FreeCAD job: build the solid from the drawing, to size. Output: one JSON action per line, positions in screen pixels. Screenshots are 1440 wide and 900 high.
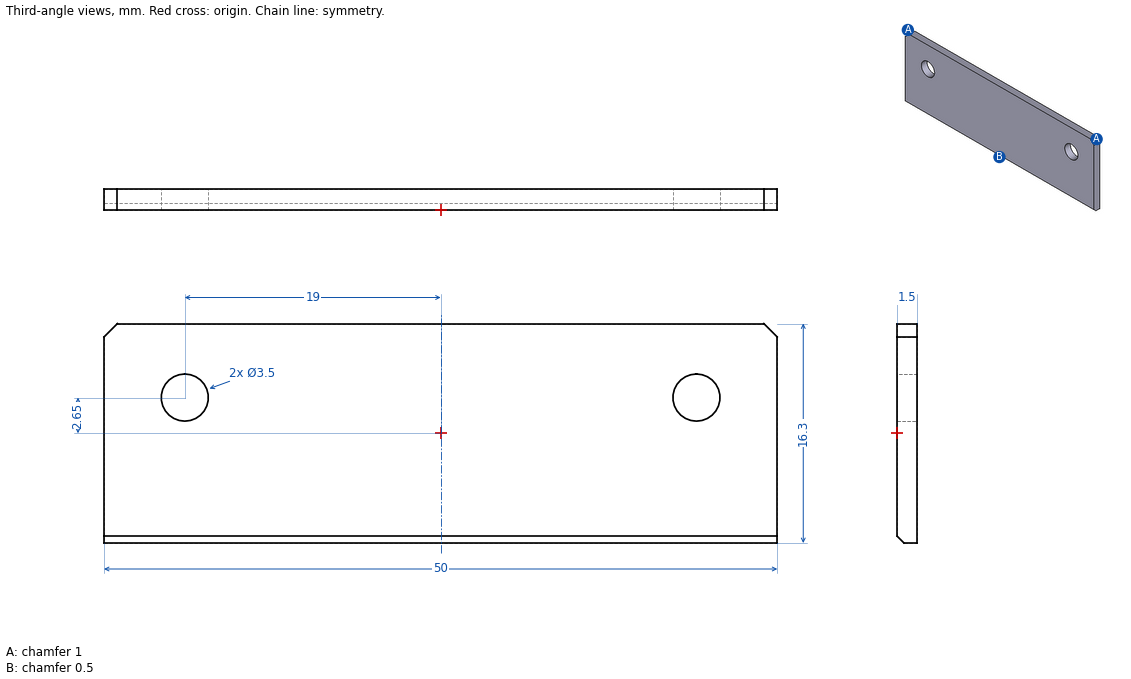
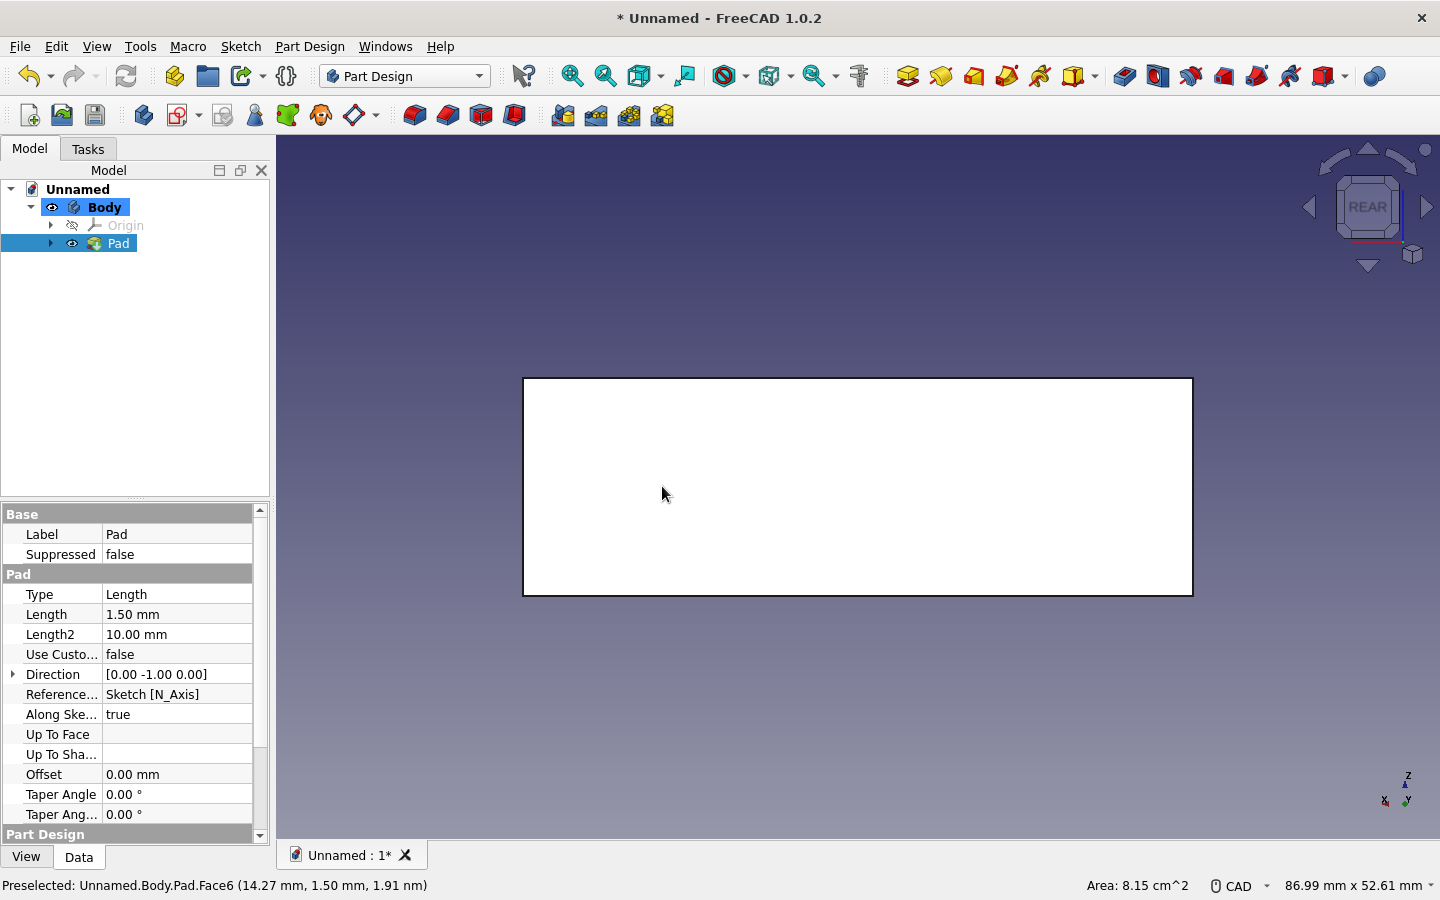
{"action": "left_click", "coordinate": [176, 116]}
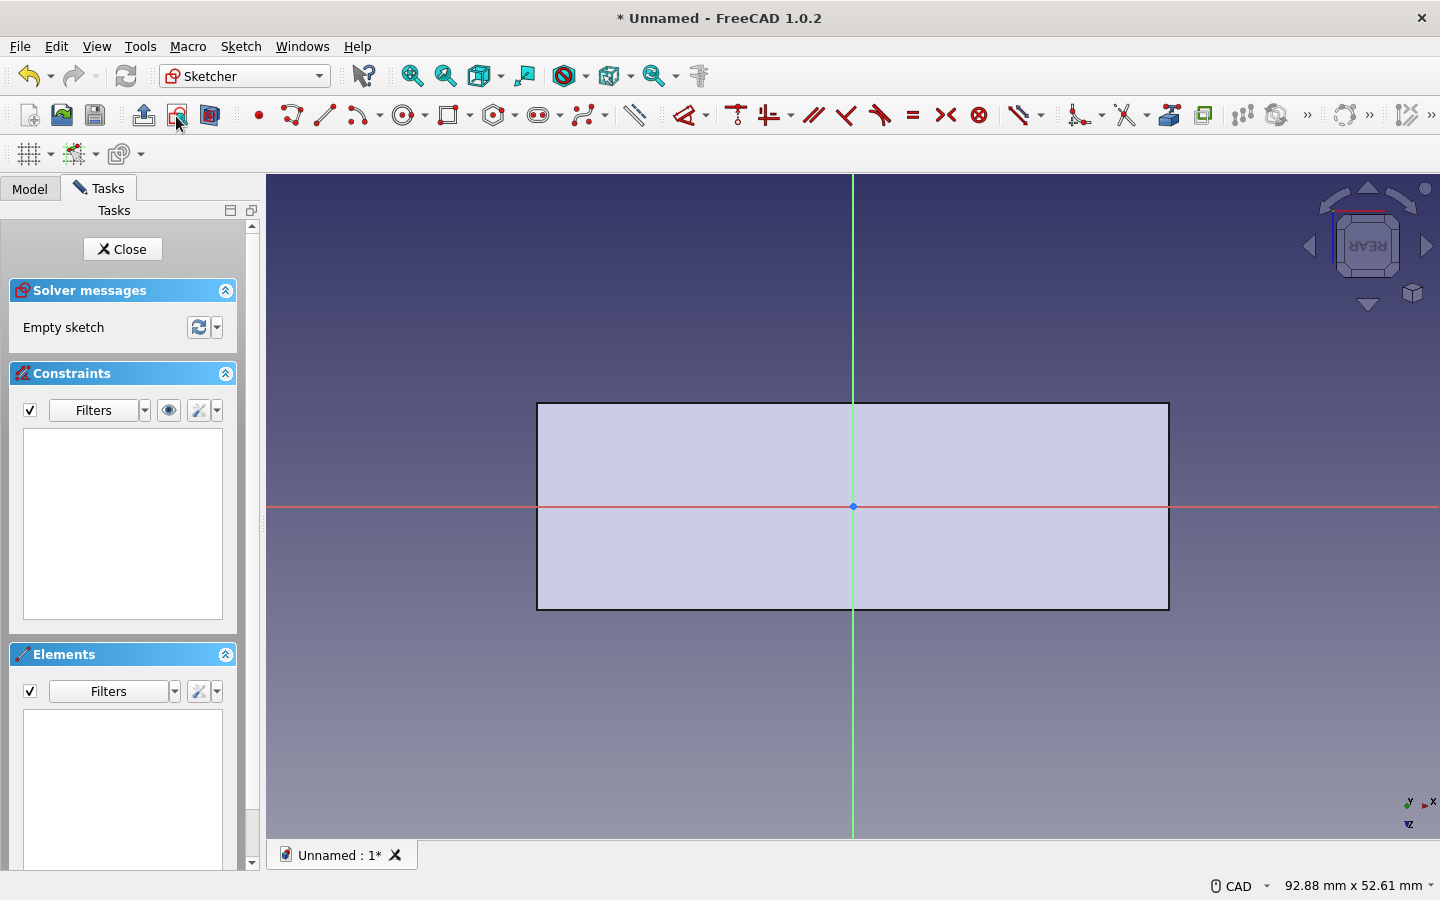
{"action": "left_click", "coordinate": [402, 116]}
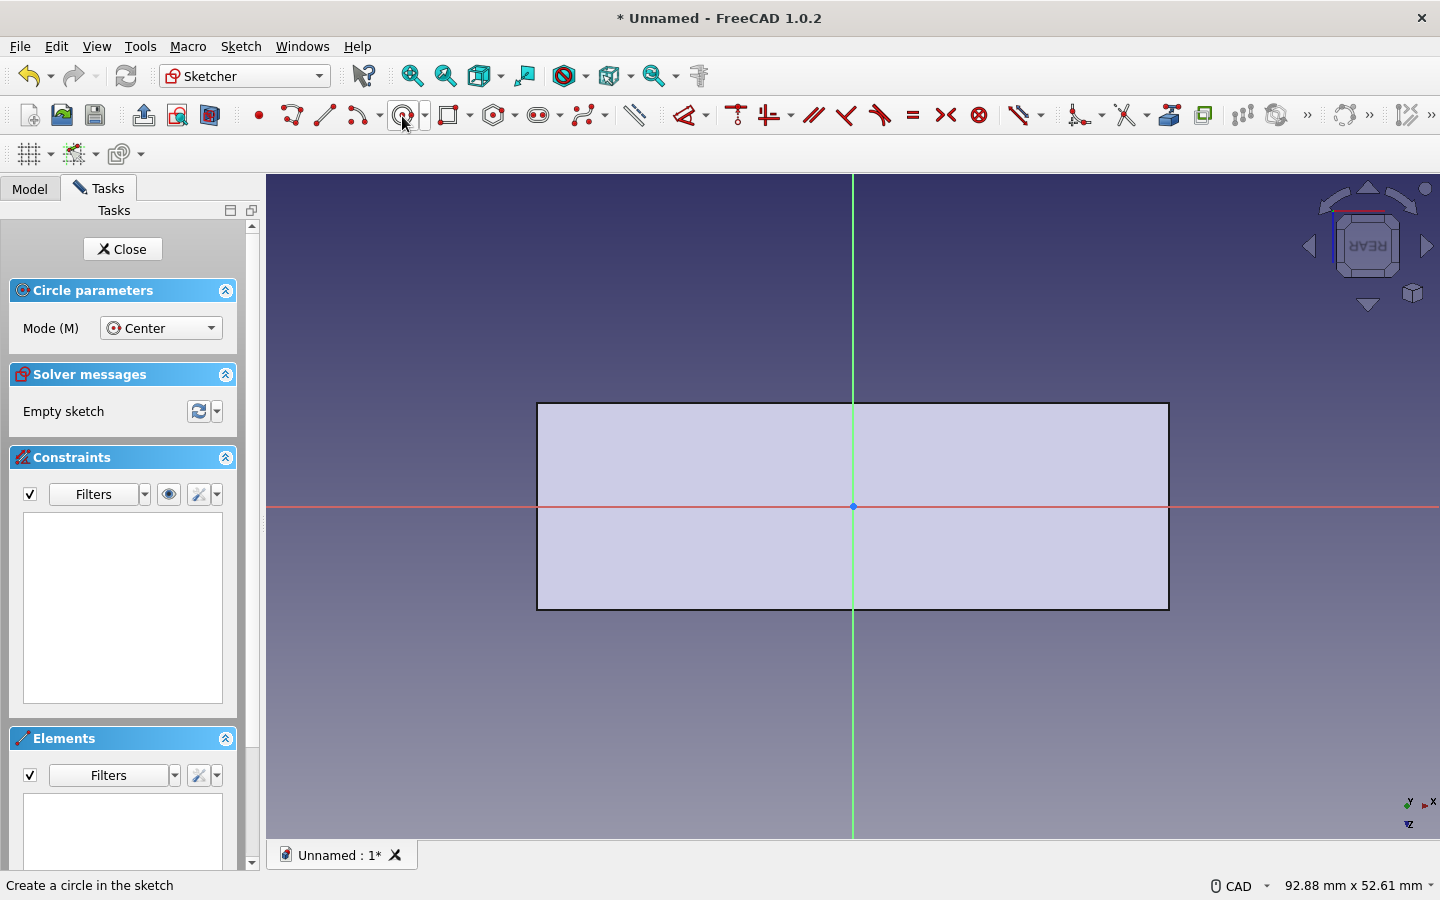
{"action": "left_click", "coordinate": [613, 540]}
{"action": "mouse_move", "coordinate": [628, 524]}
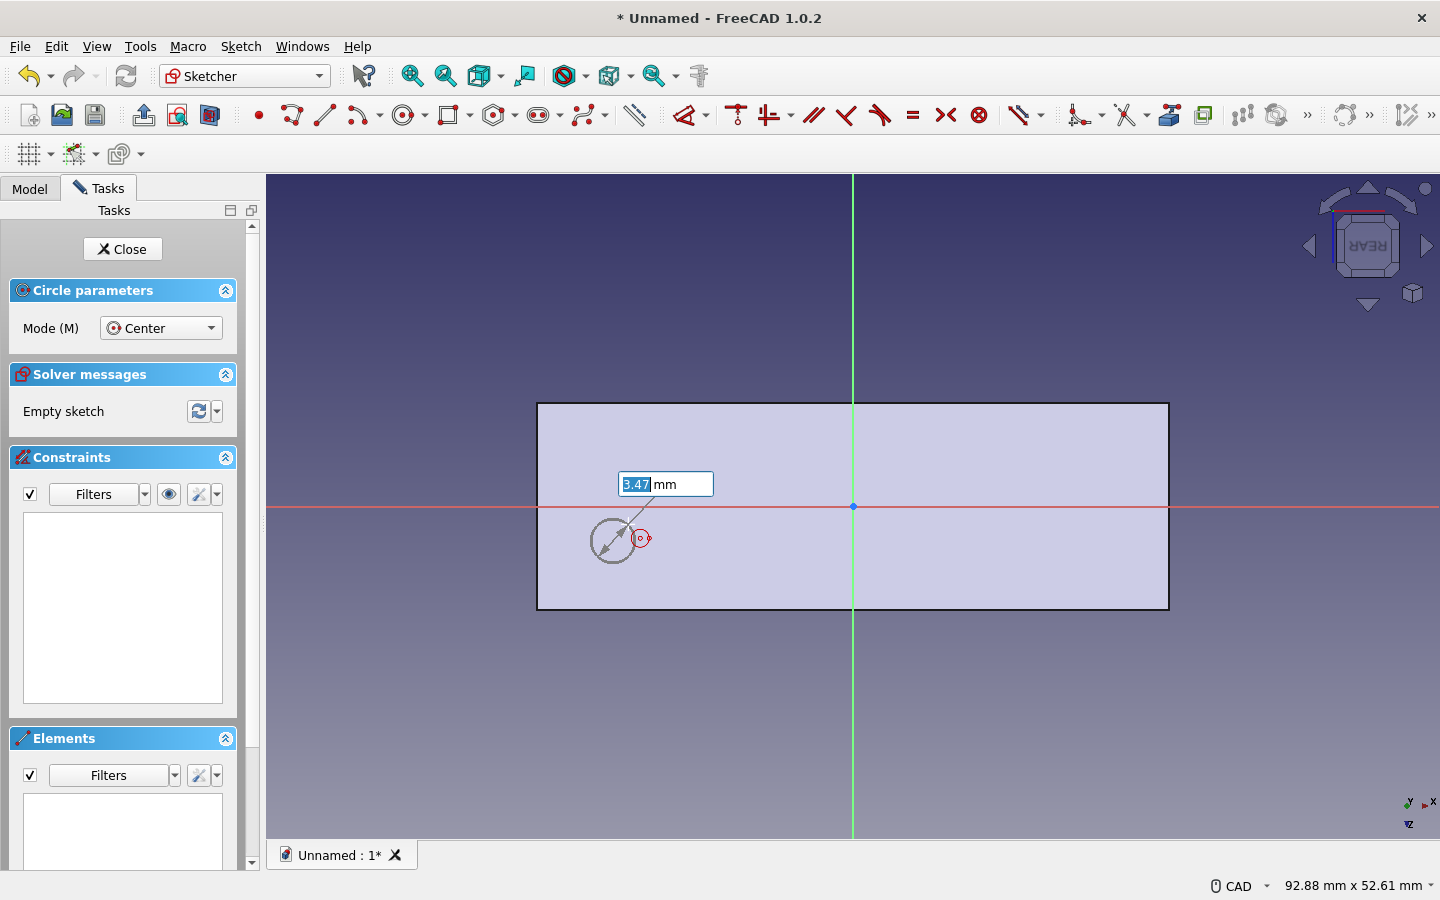
{"action": "type", "text": "3.5"}
{"action": "key", "text": "Return"}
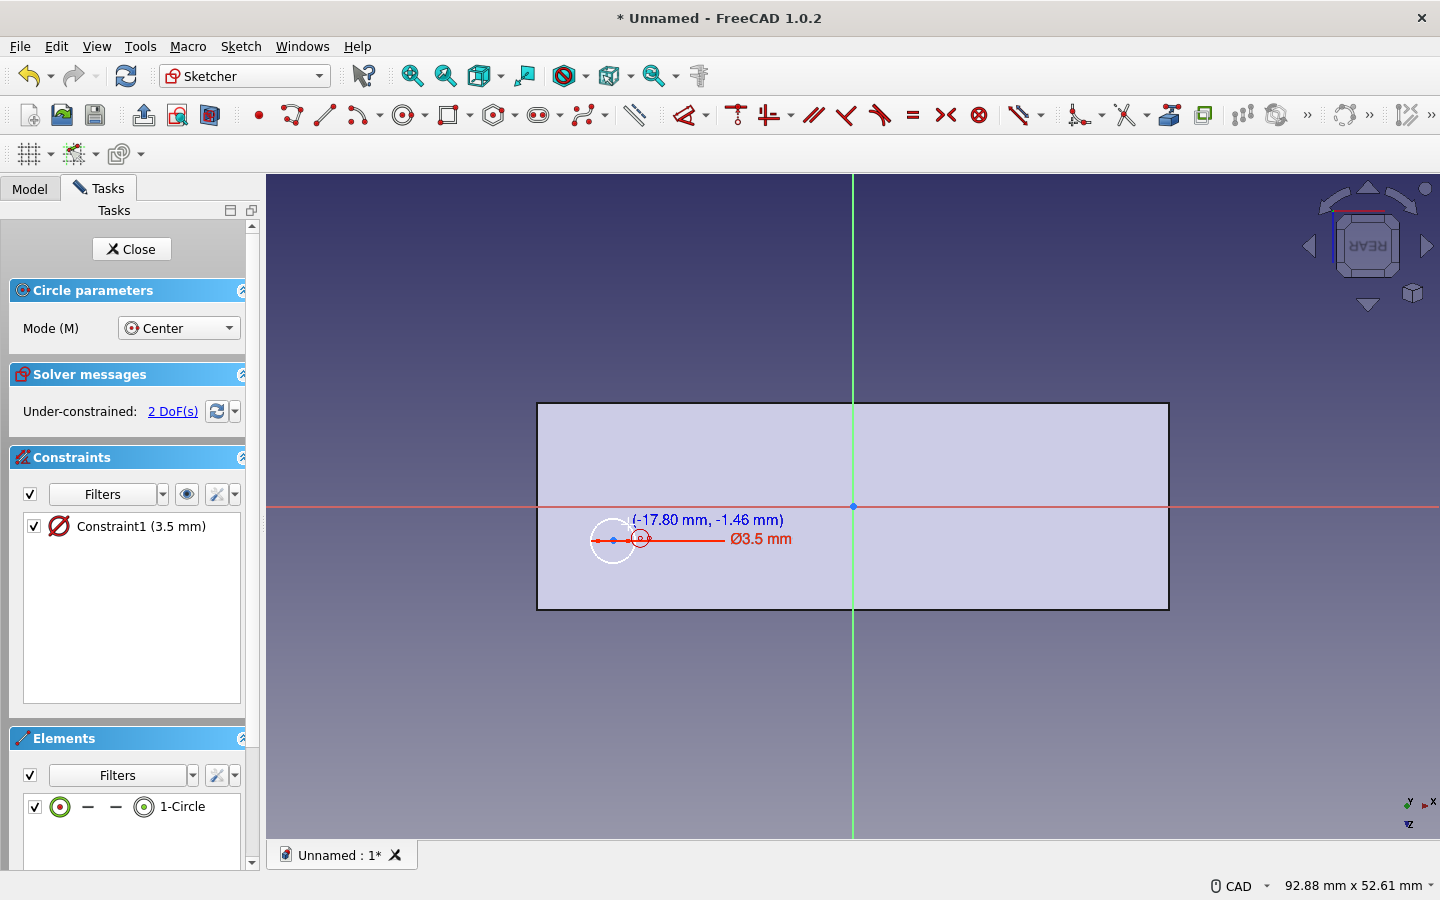
{"action": "left_click", "coordinate": [1093, 540]}
{"action": "mouse_move", "coordinate": [1109, 524]}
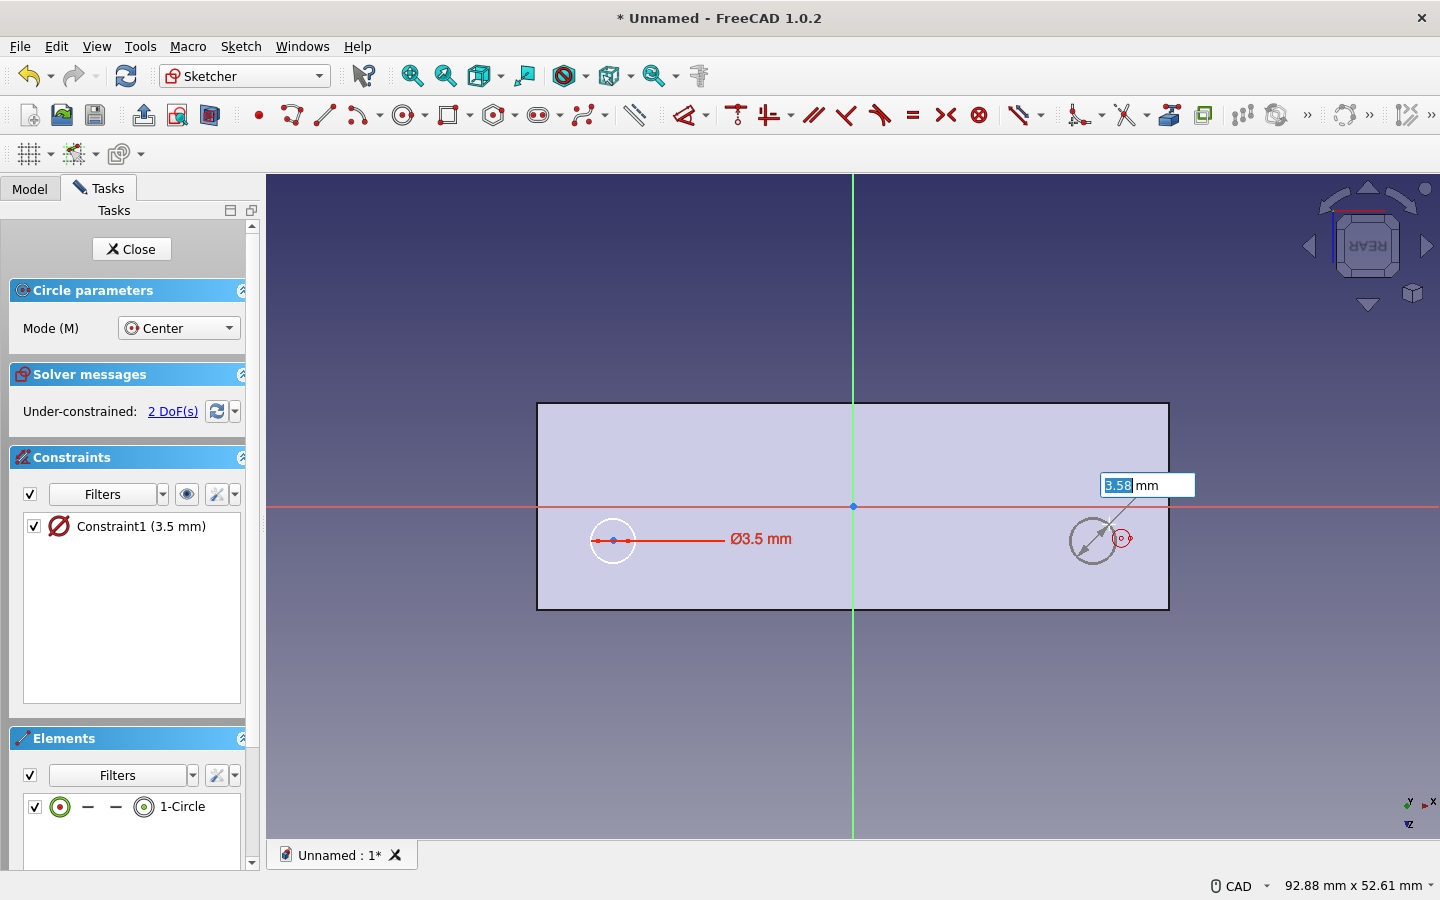
{"action": "type", "text": "3.5"}
{"action": "key", "text": "Return"}
{"action": "key", "text": "Escape"}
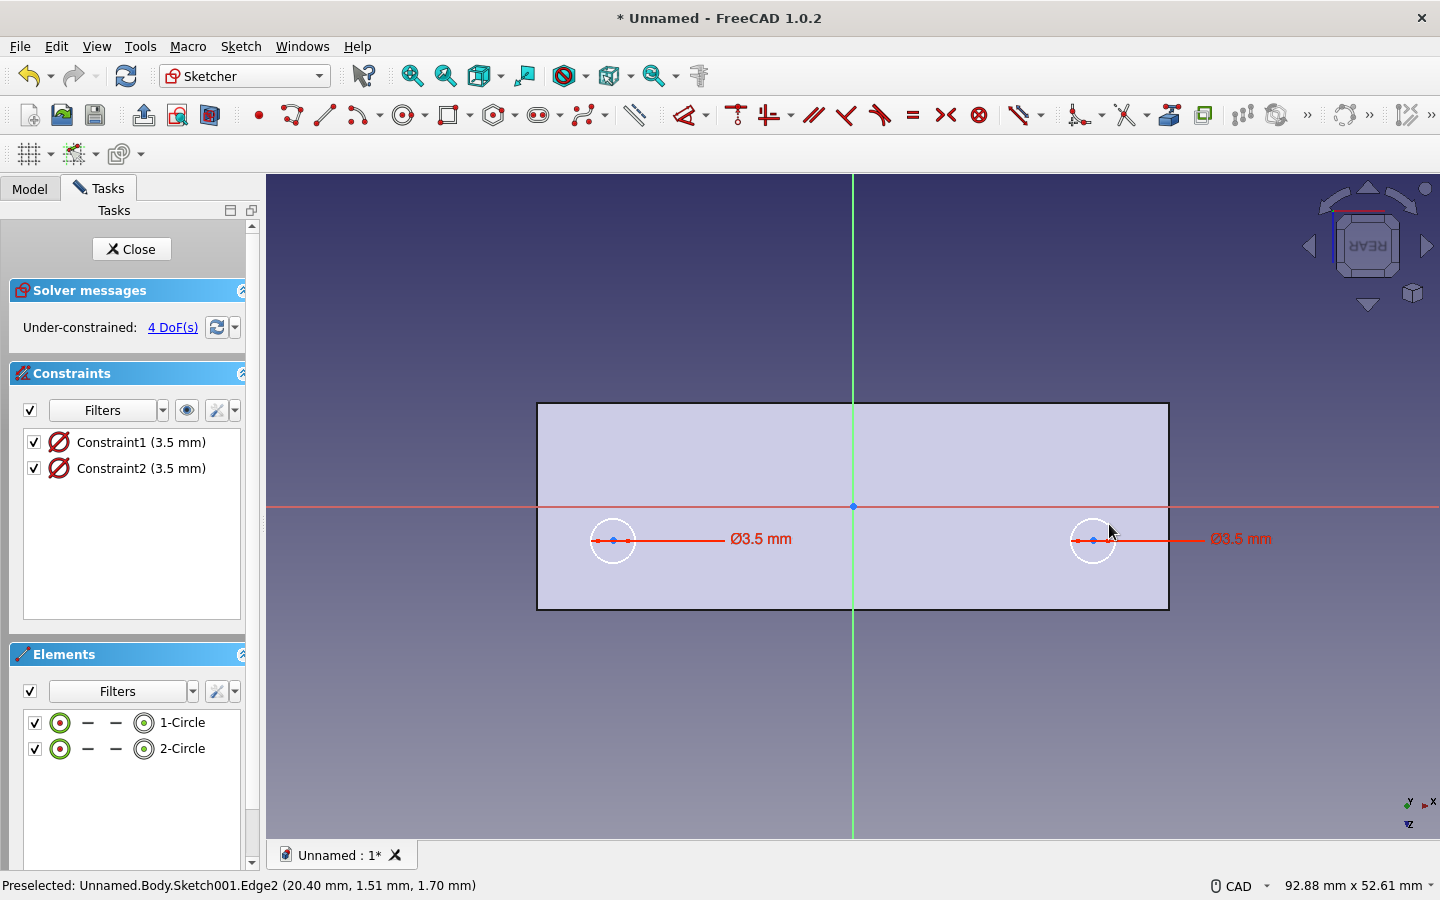
{"action": "left_click", "coordinate": [613, 541]}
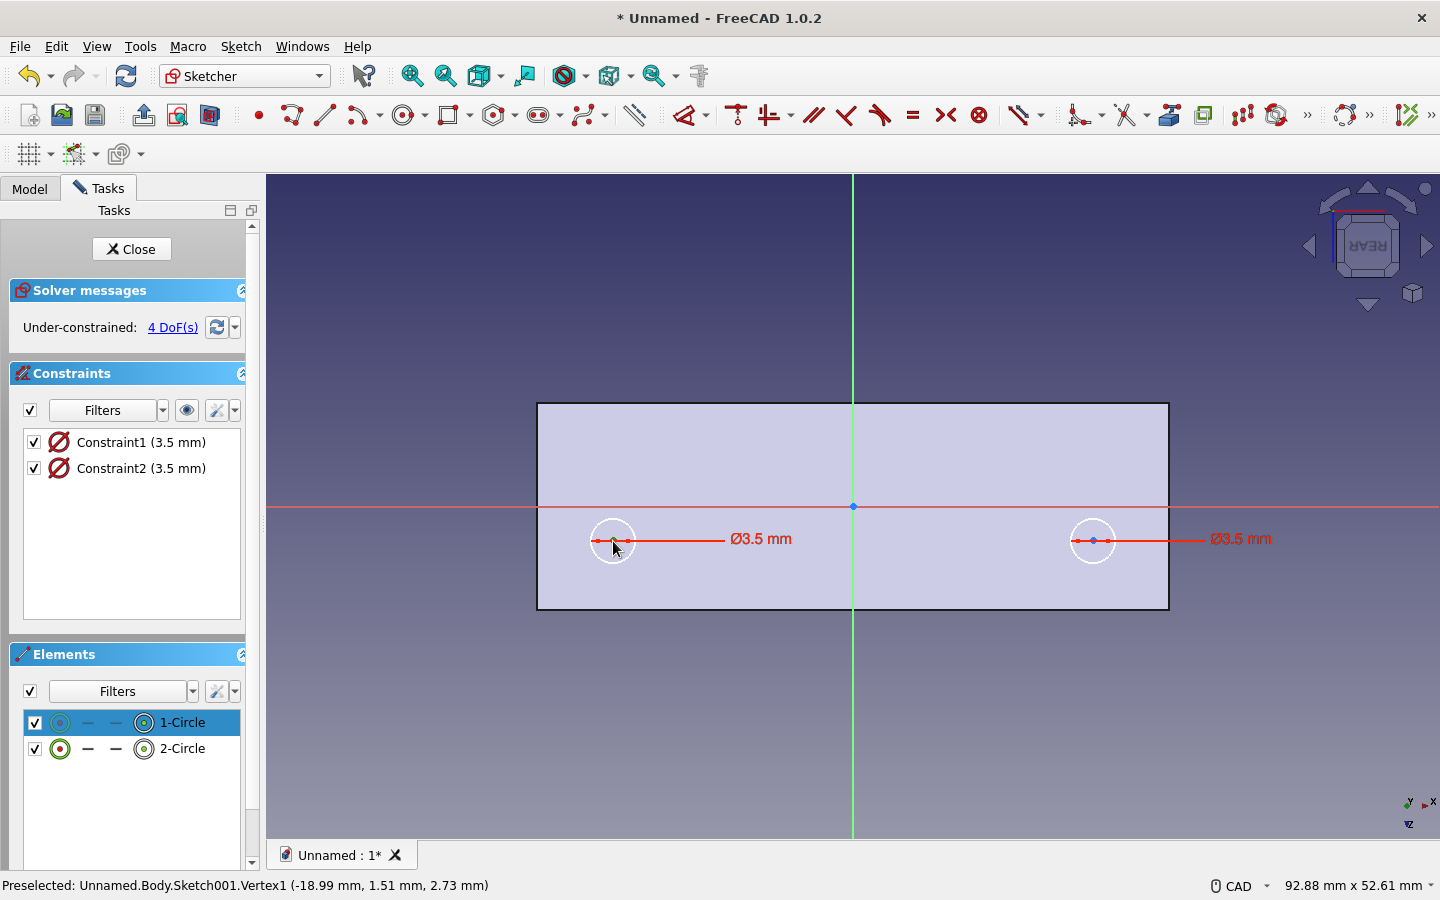
{"action": "left_click", "coordinate": [1093, 541]}